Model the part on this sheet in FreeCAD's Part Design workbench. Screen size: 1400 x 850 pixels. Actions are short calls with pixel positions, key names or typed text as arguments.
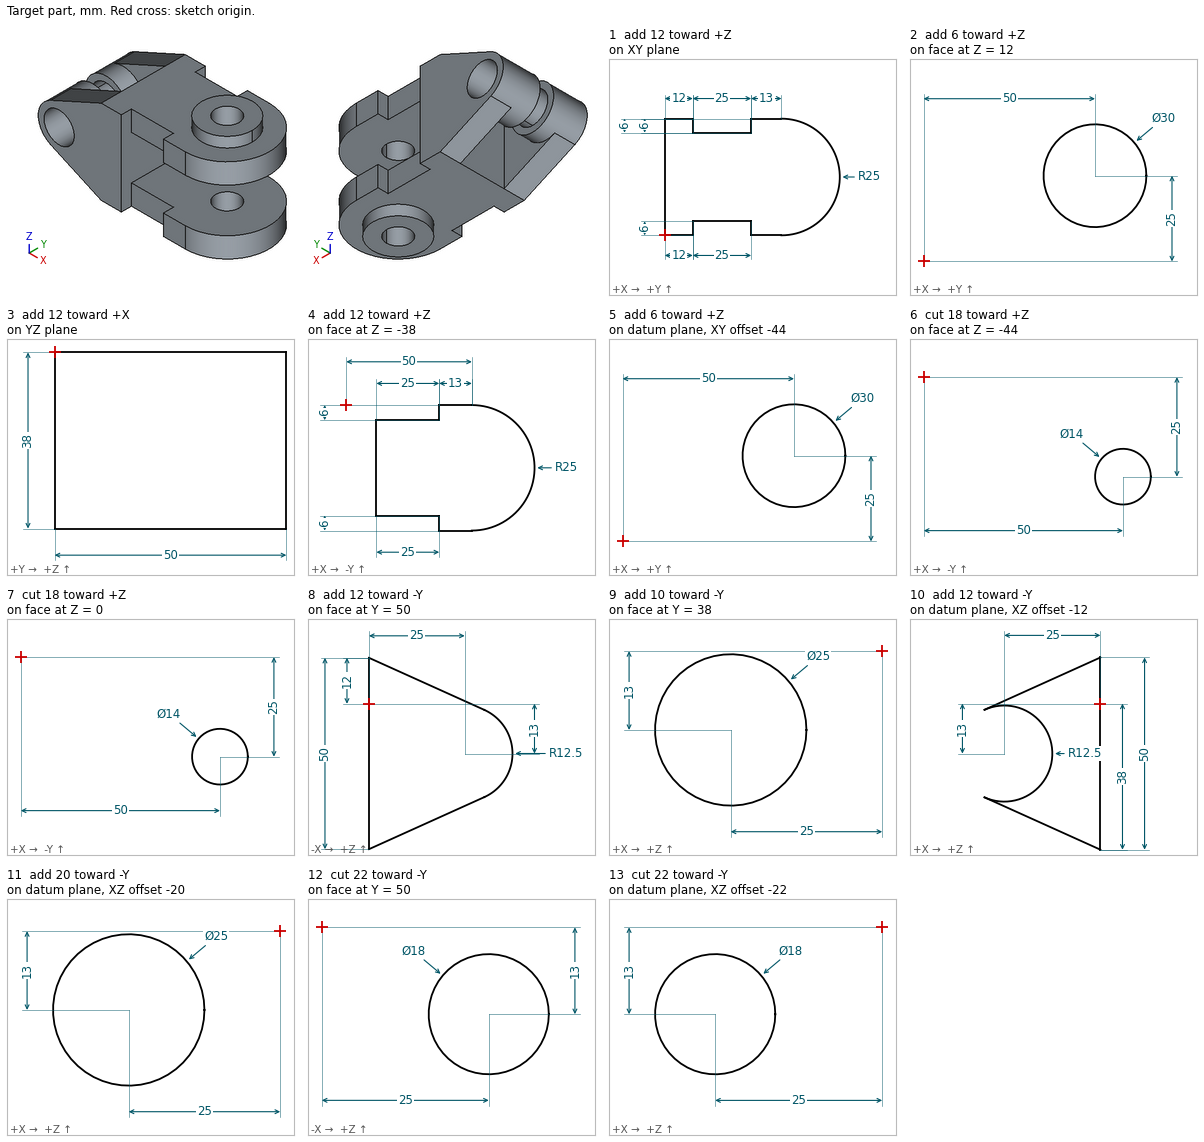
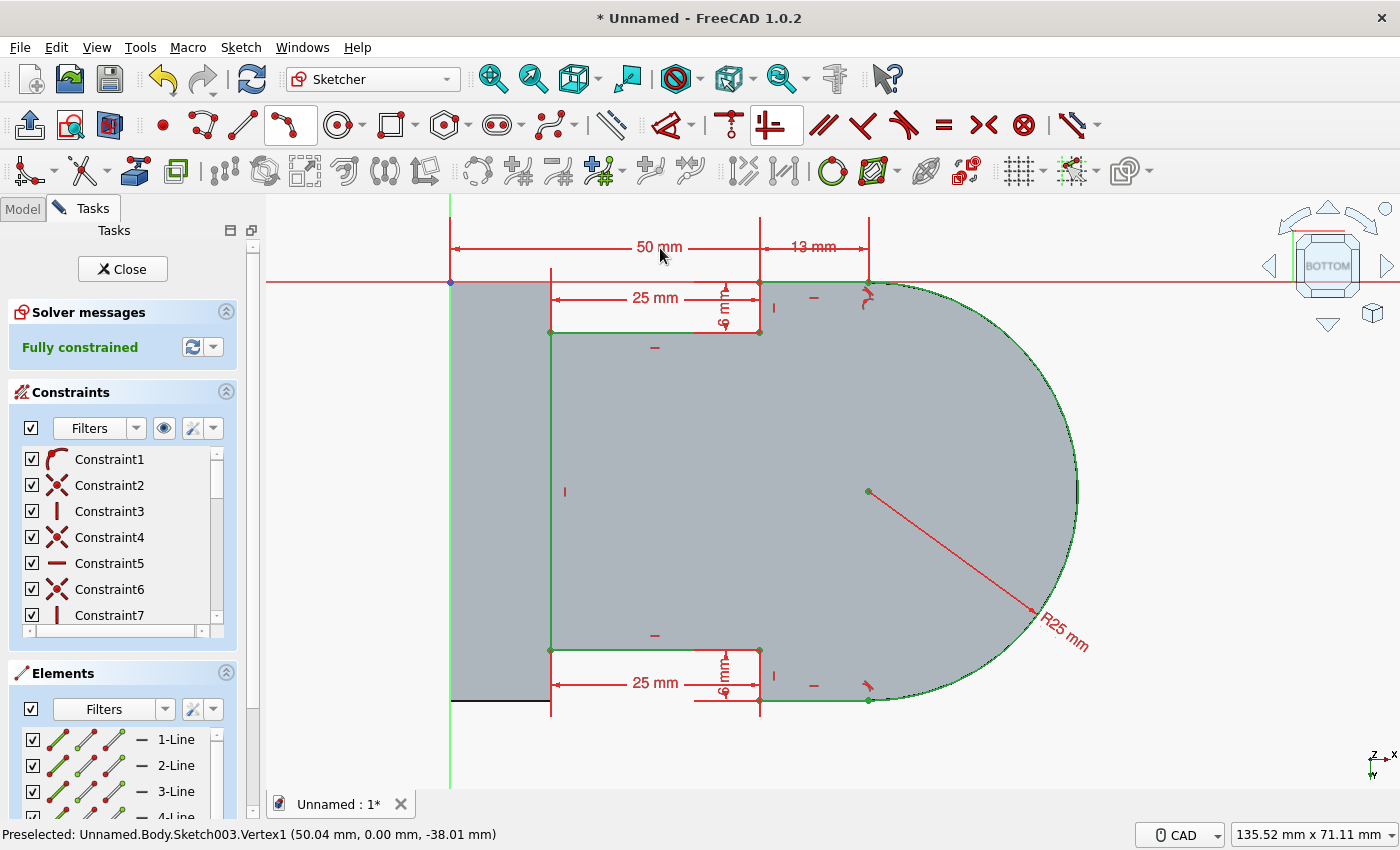
click(123, 269)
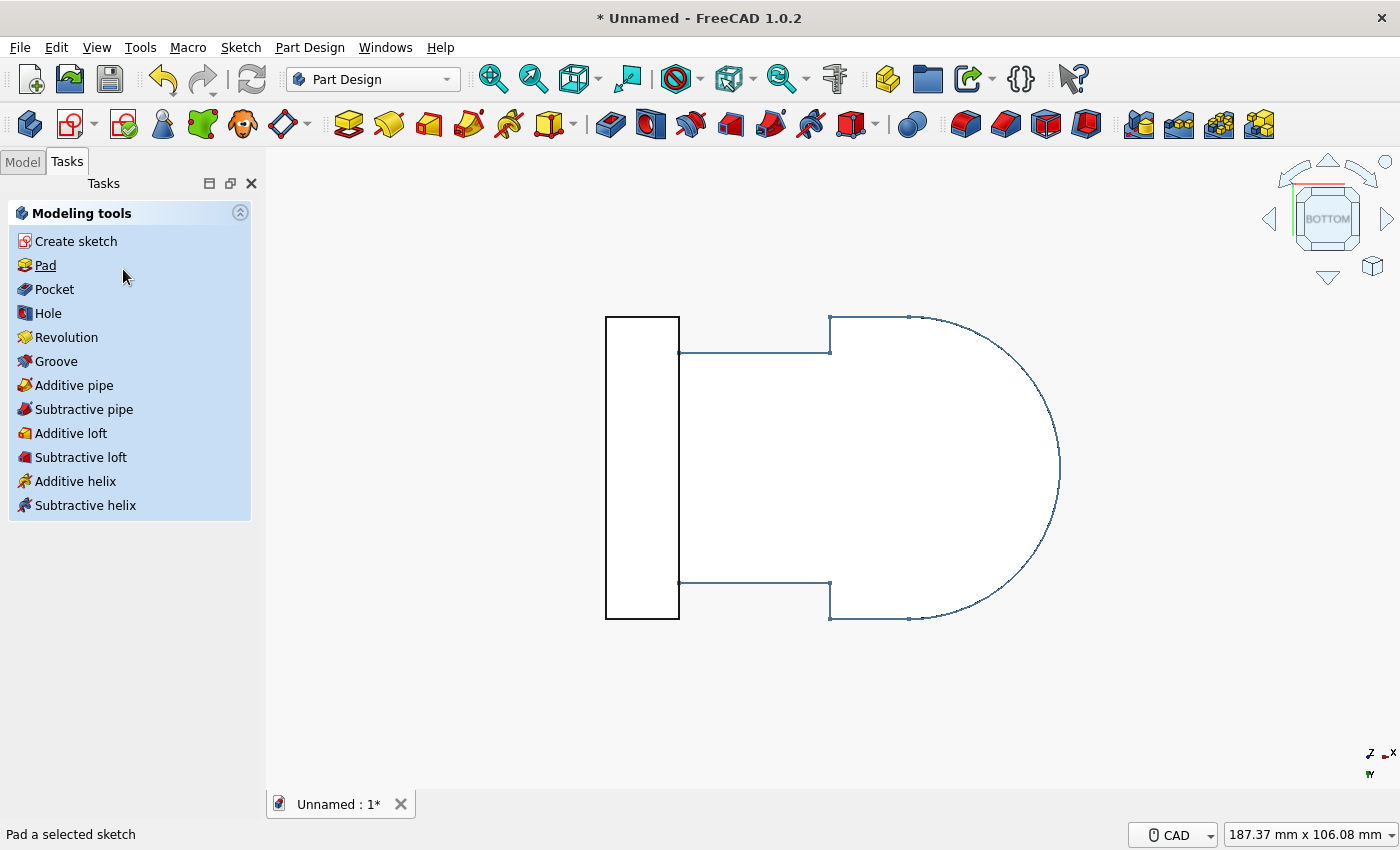
click(350, 124)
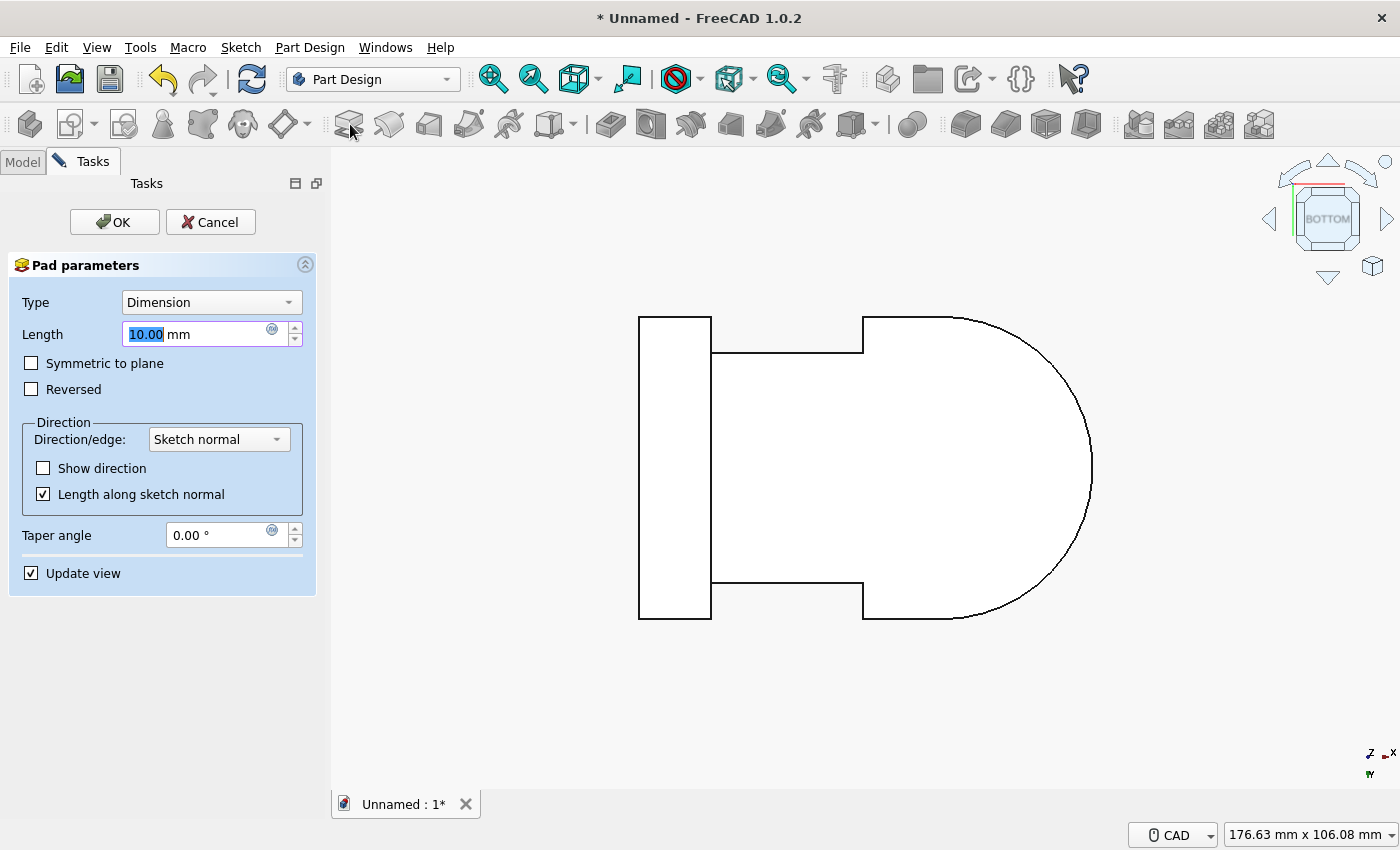
text(12)
key(Tab)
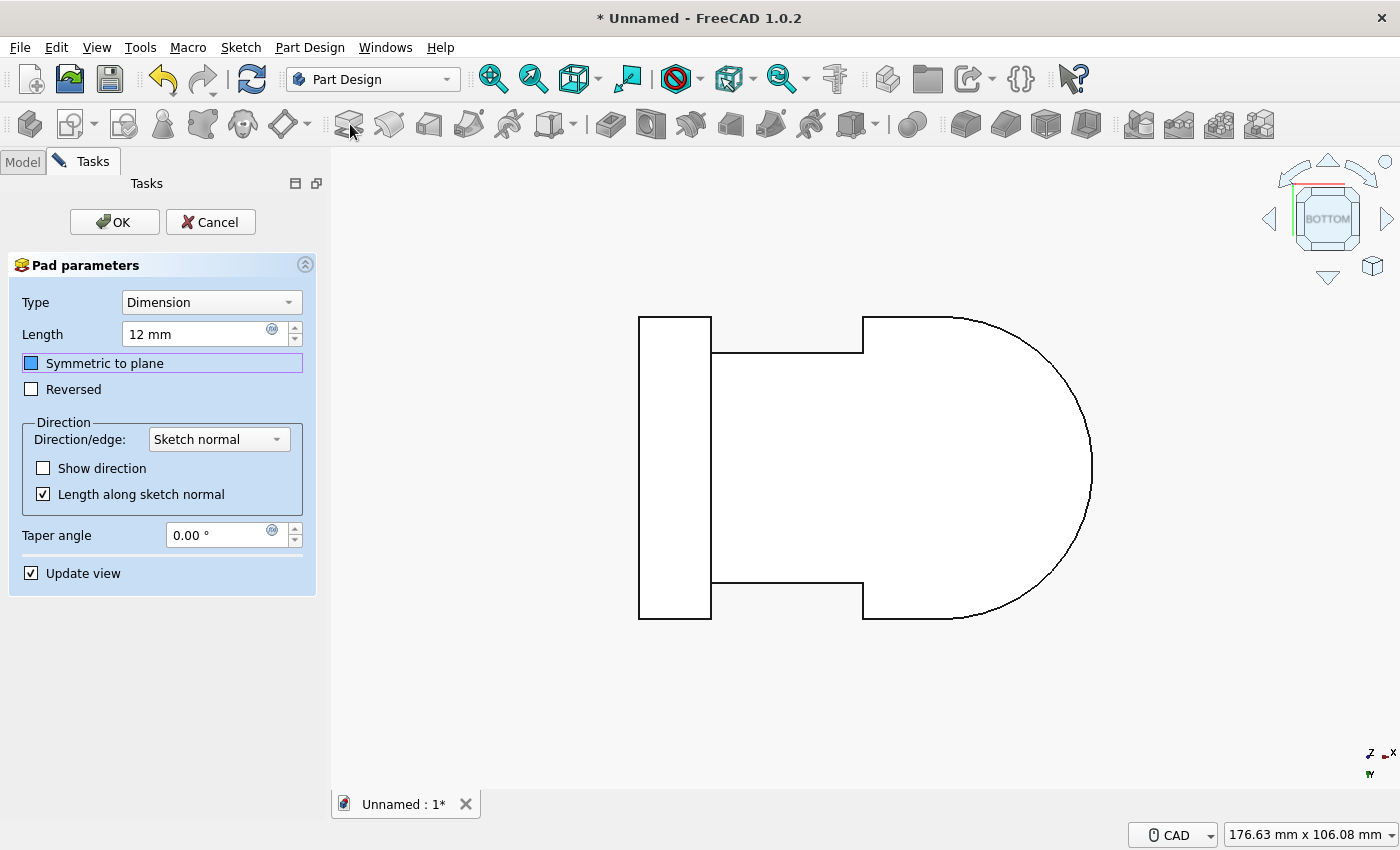
click(30, 389)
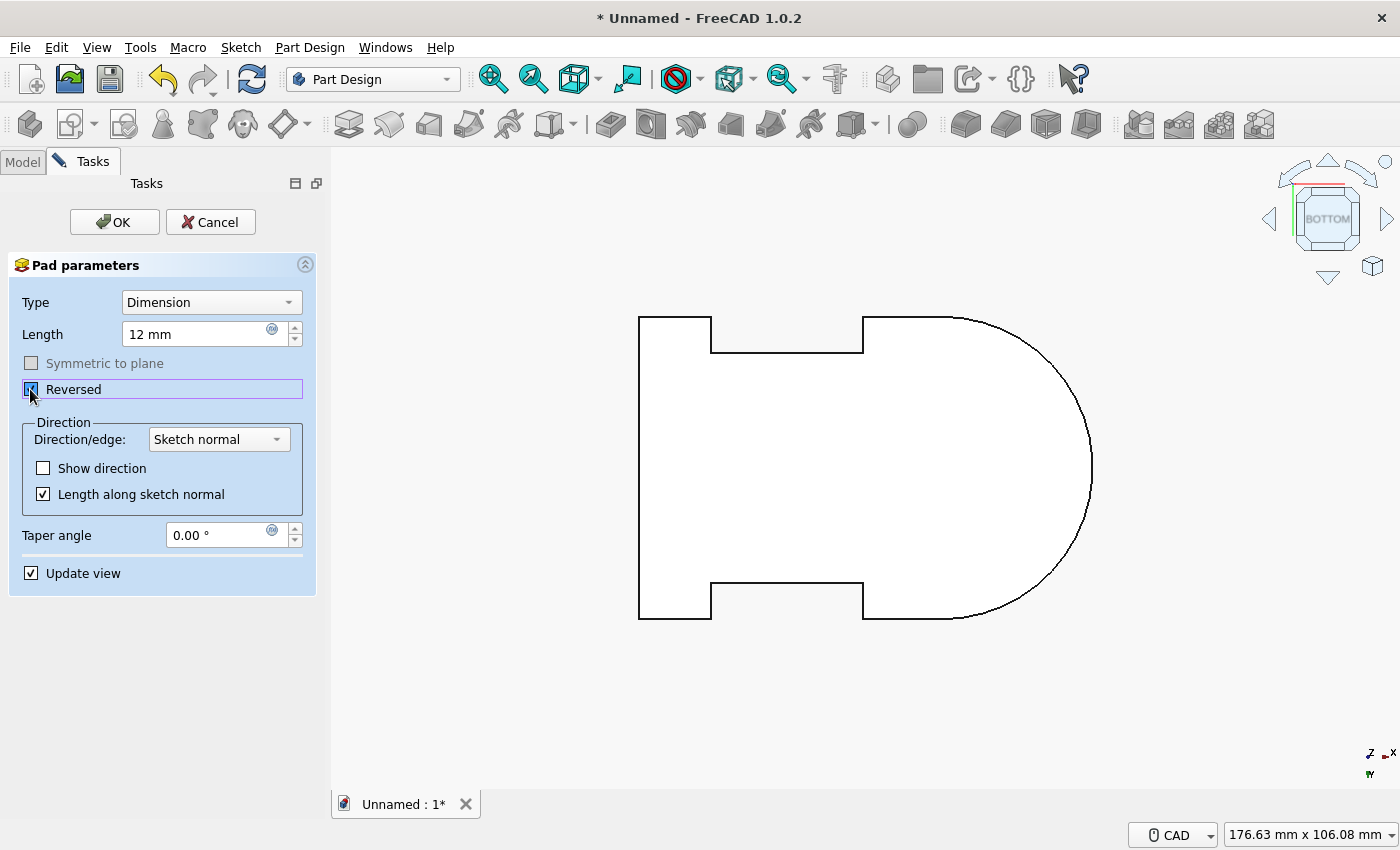
click(115, 222)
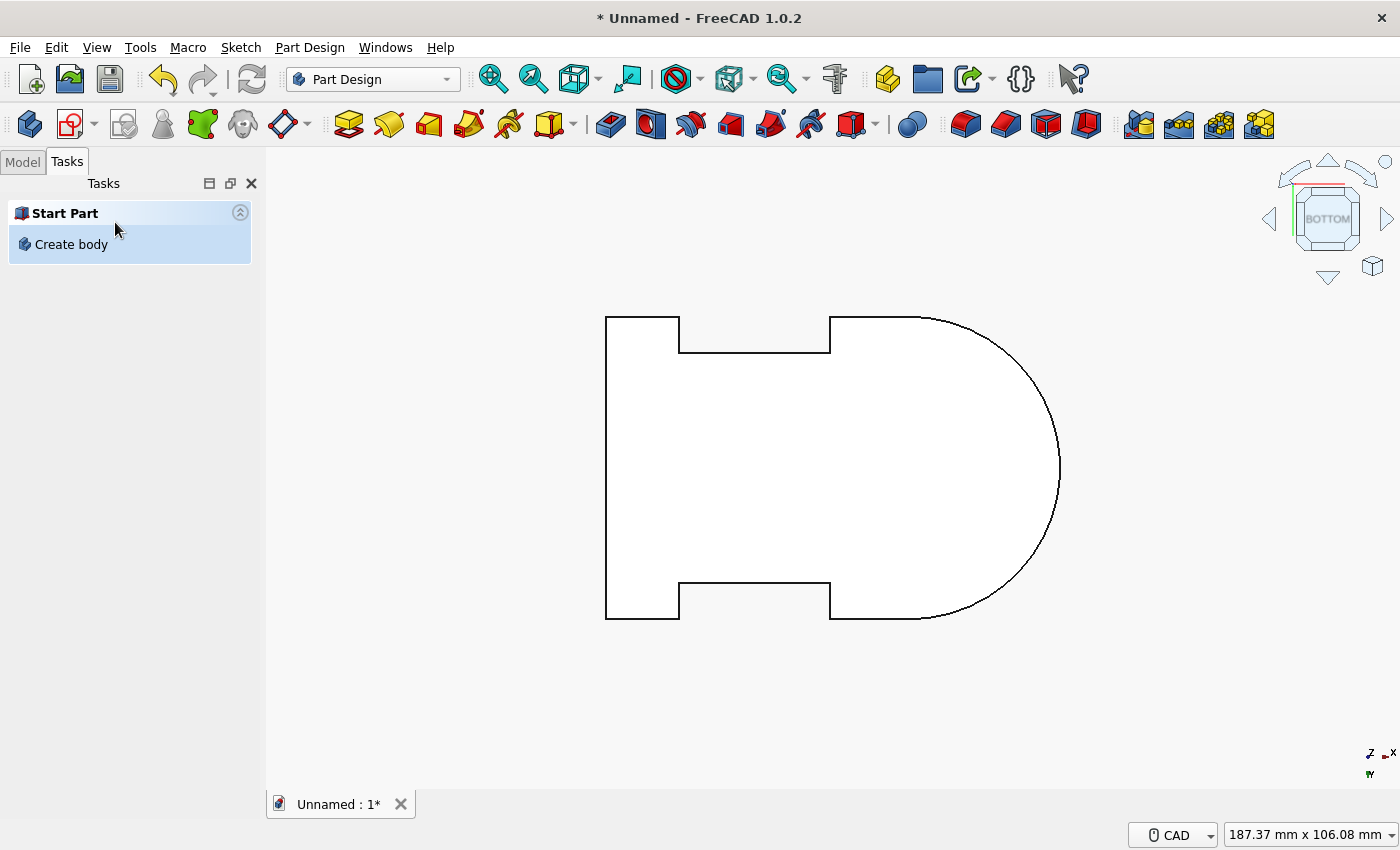
click(23, 161)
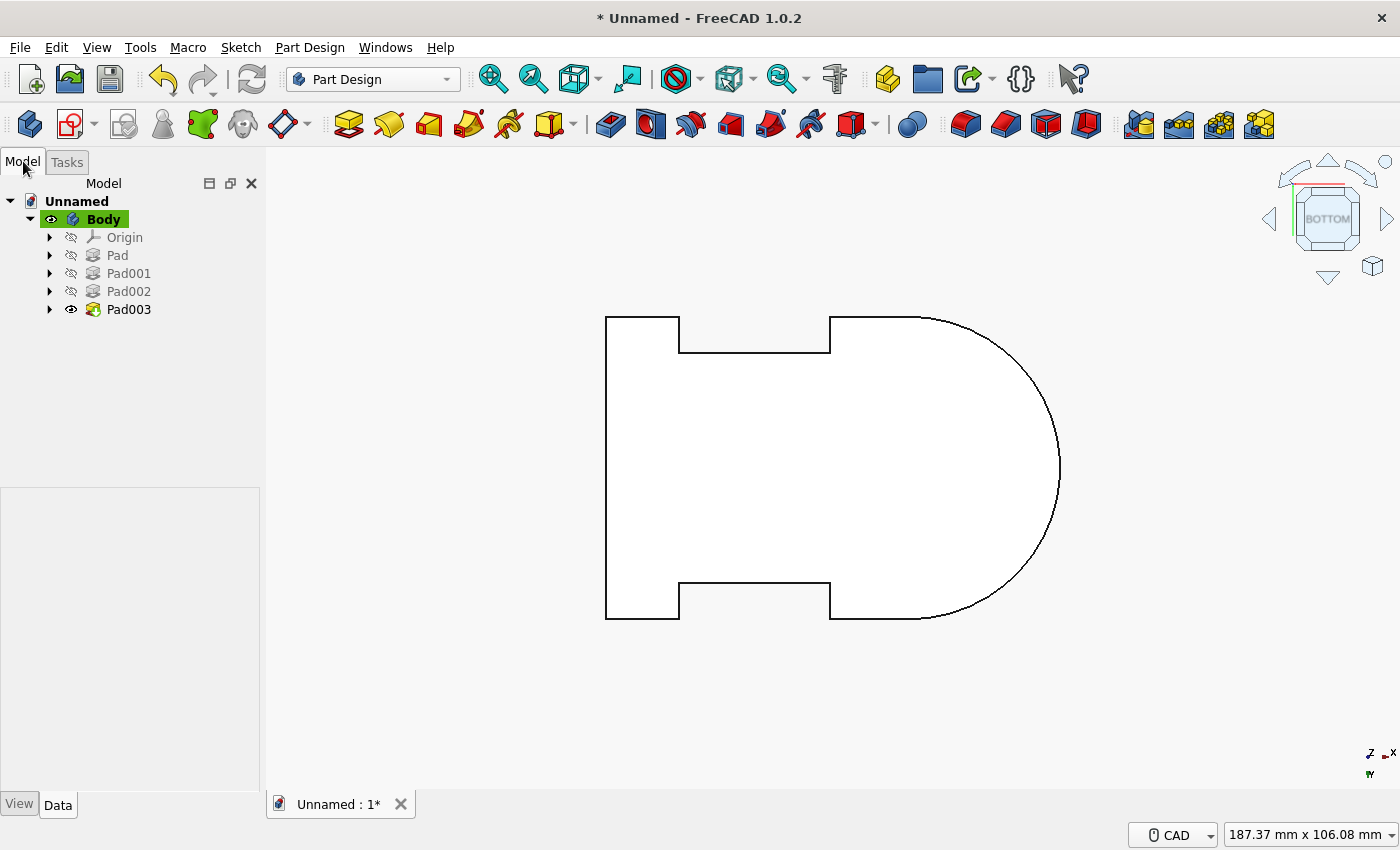
click(50, 237)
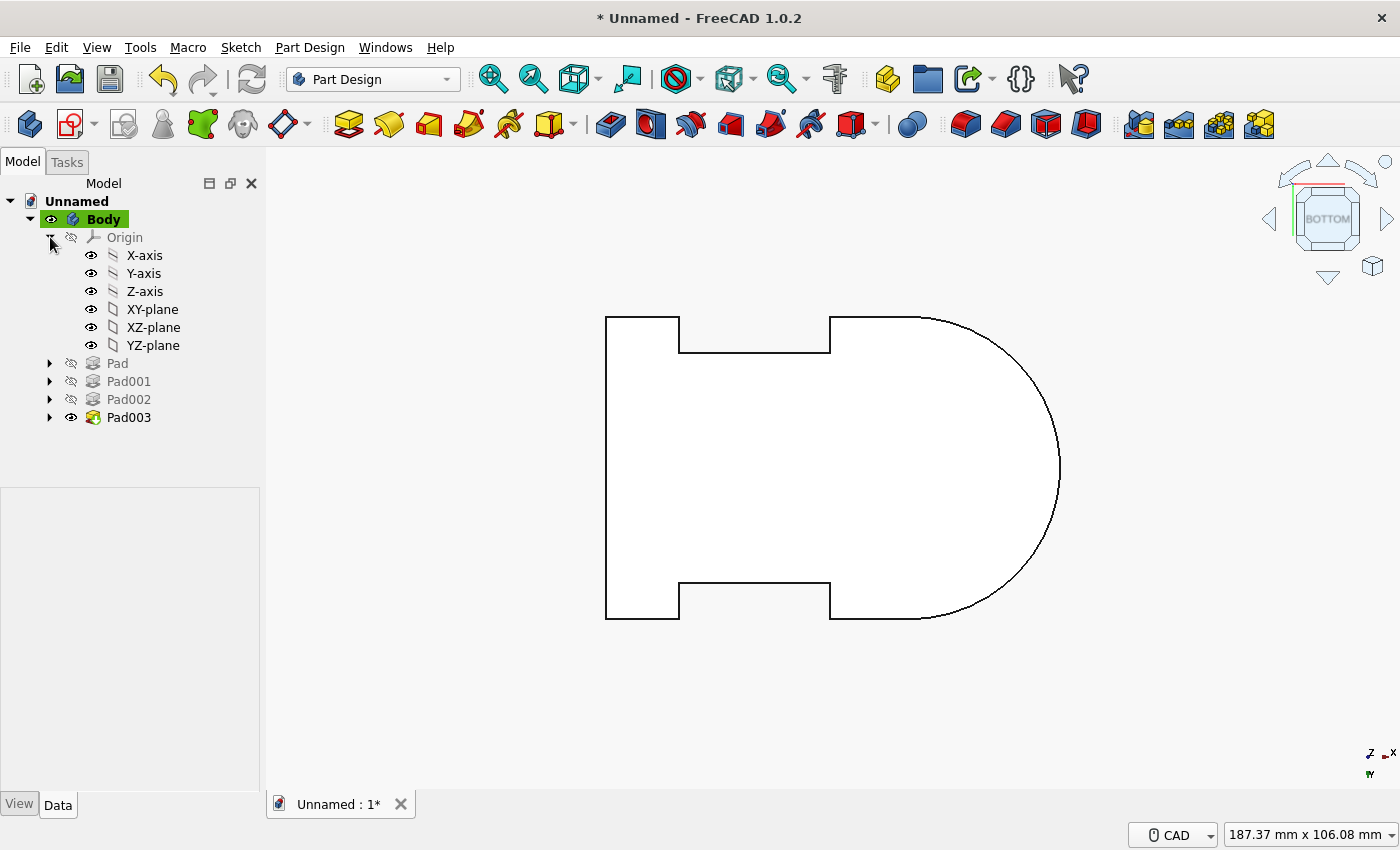
click(136, 309)